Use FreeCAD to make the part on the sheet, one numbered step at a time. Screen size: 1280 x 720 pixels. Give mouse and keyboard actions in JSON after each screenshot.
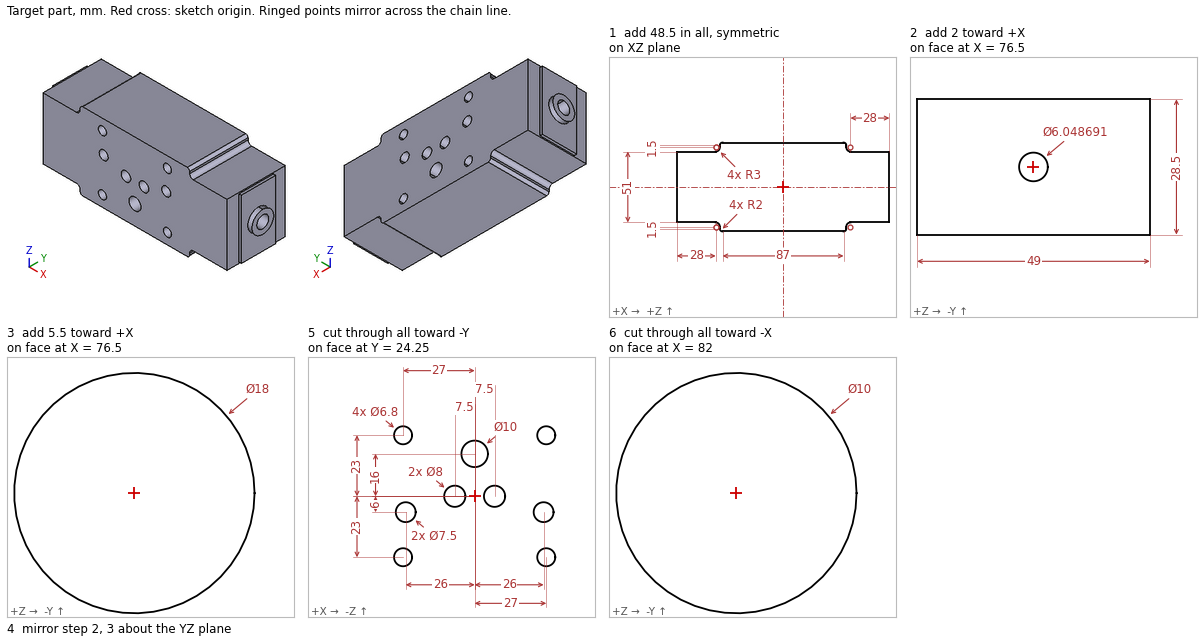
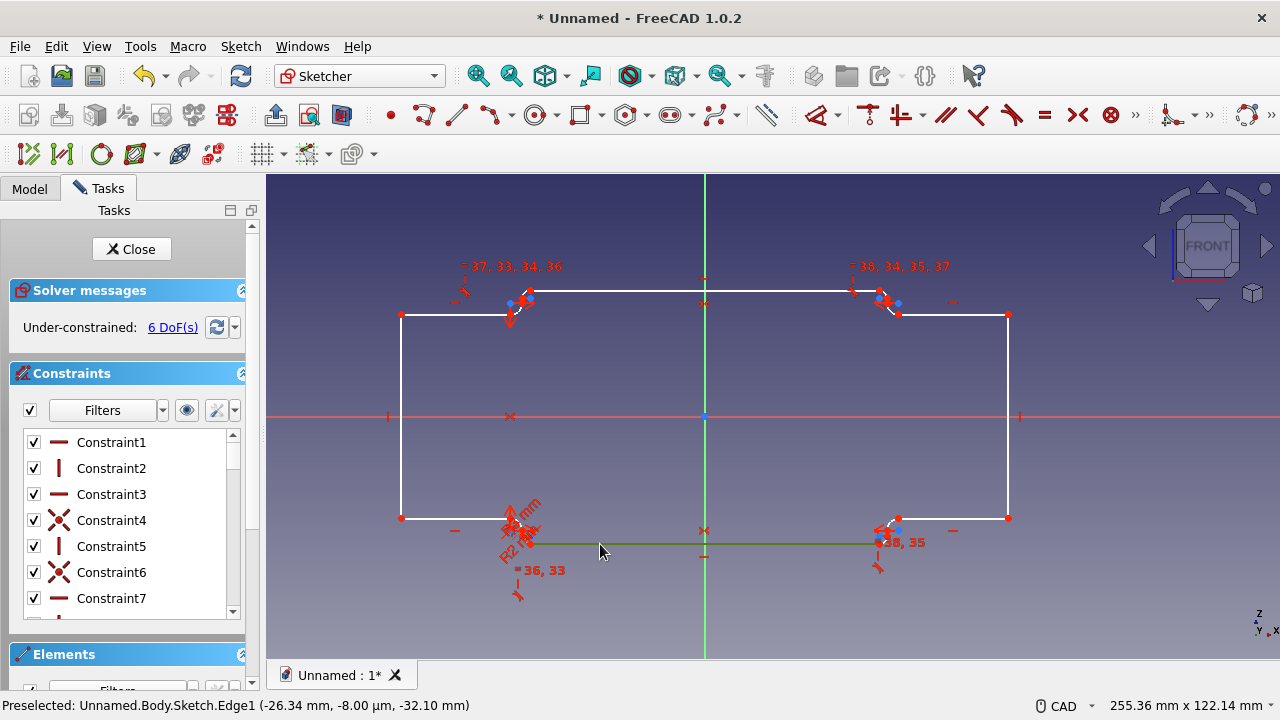
{"action": "key", "text": "l"}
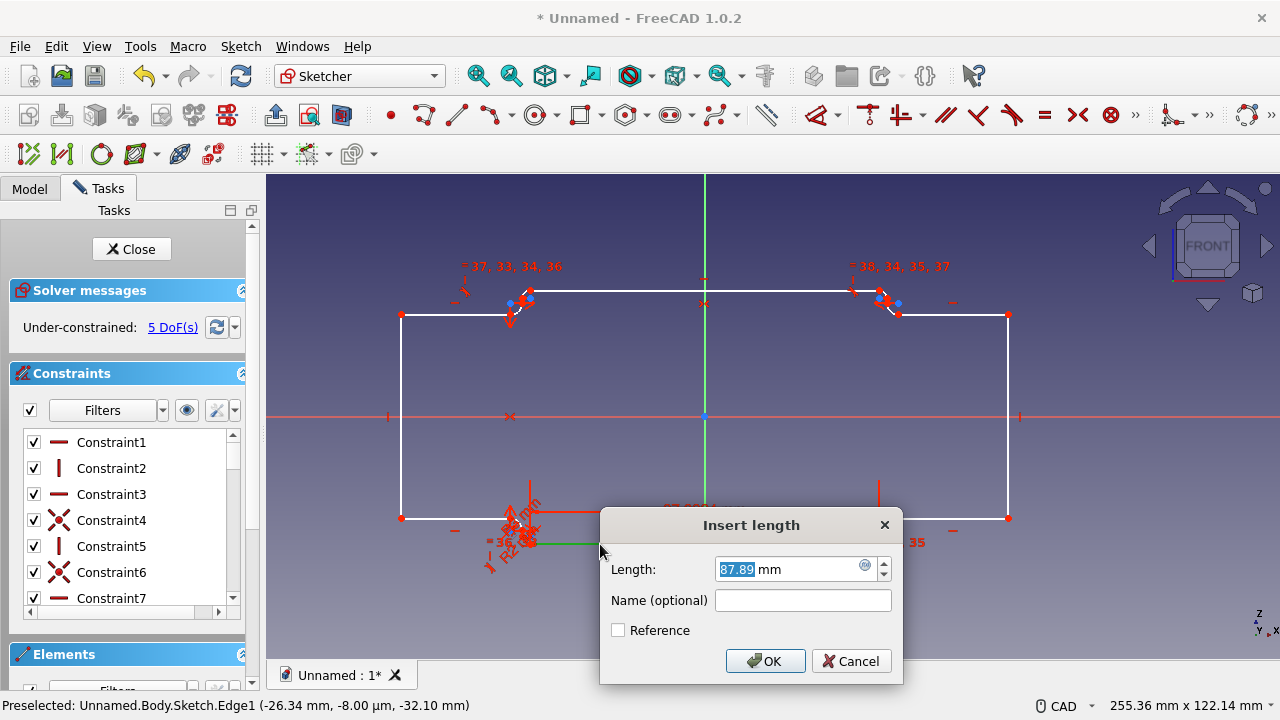
{"action": "type", "text": "87"}
{"action": "key", "text": "Return"}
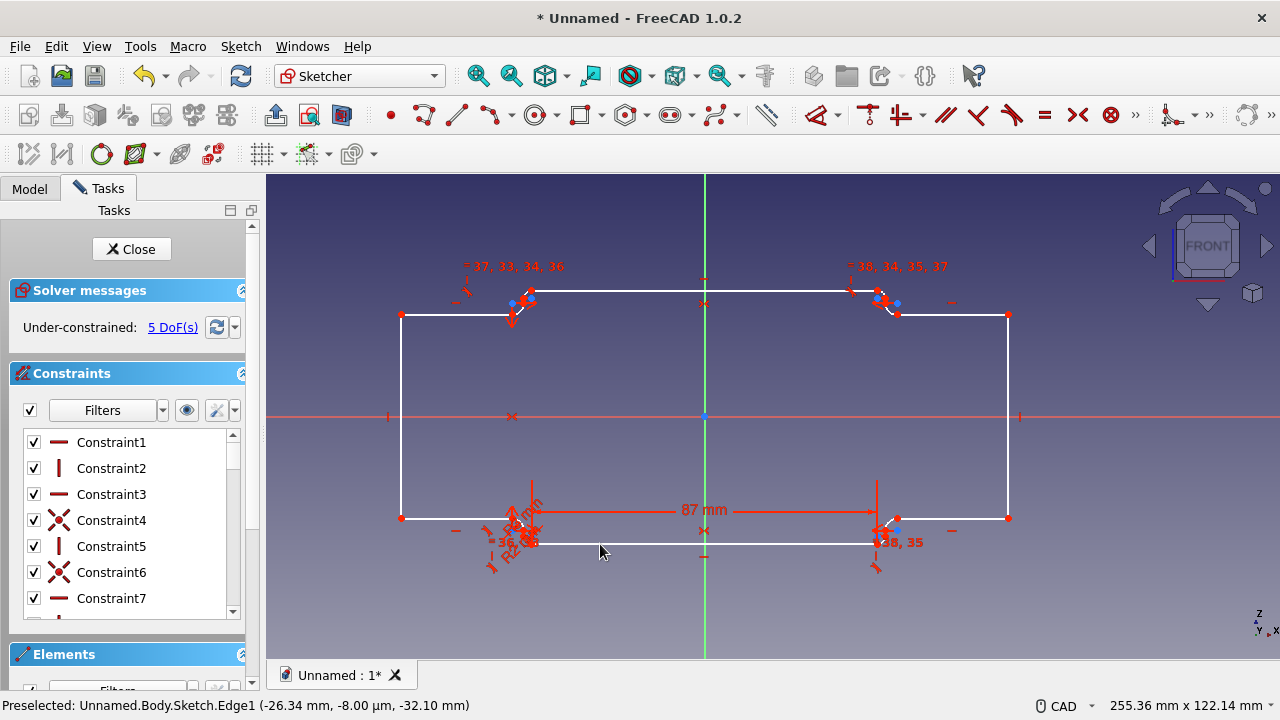
{"action": "left_click", "coordinate": [479, 519]}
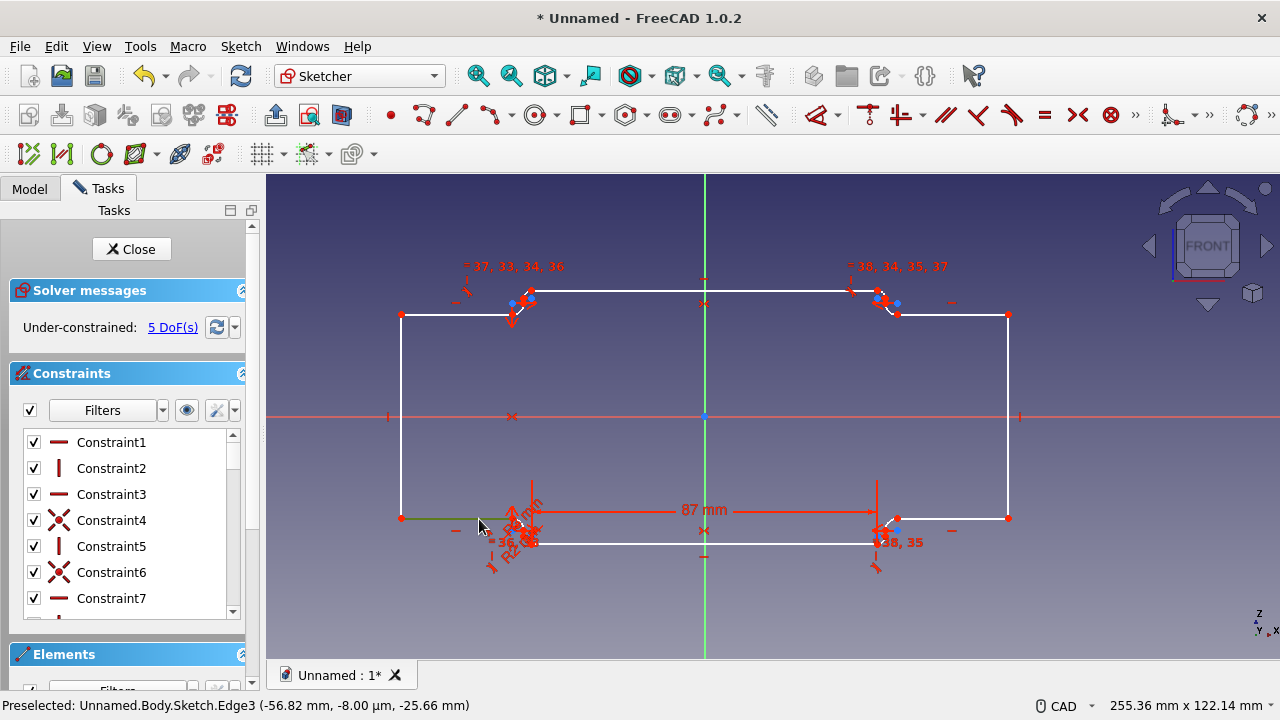
{"action": "key", "text": "l"}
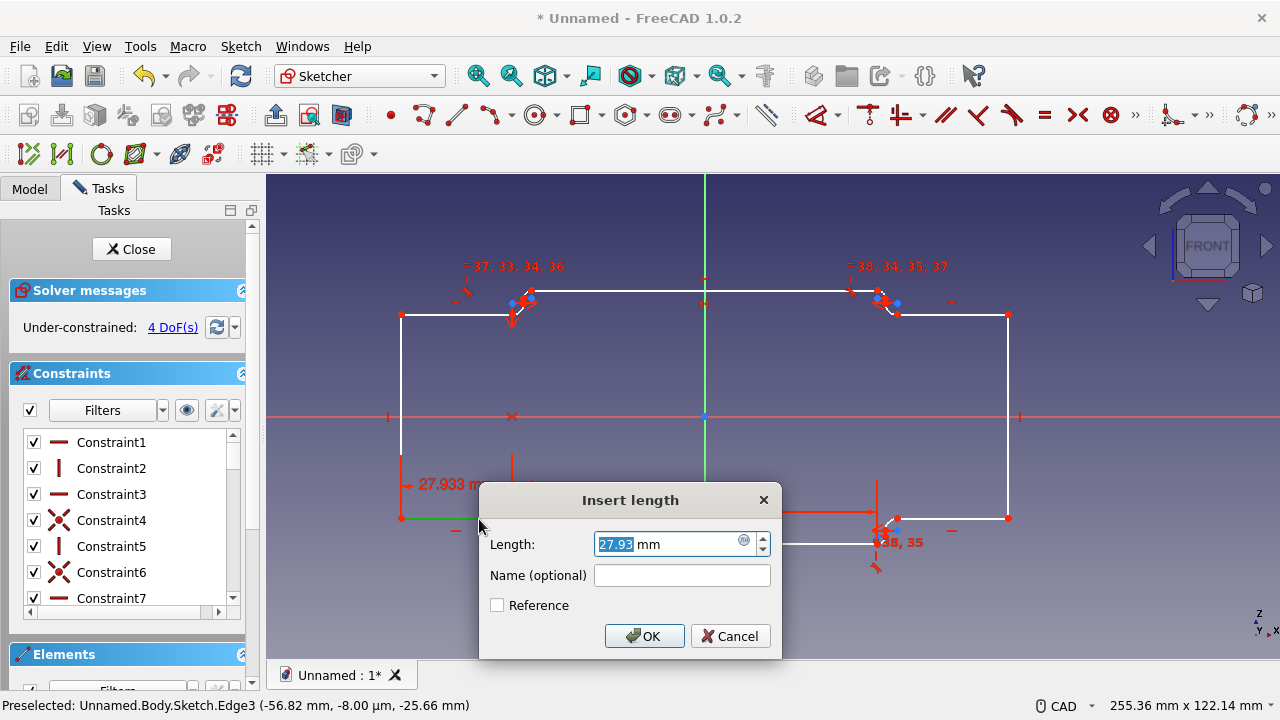
{"action": "type", "text": "28"}
{"action": "key", "text": "Return"}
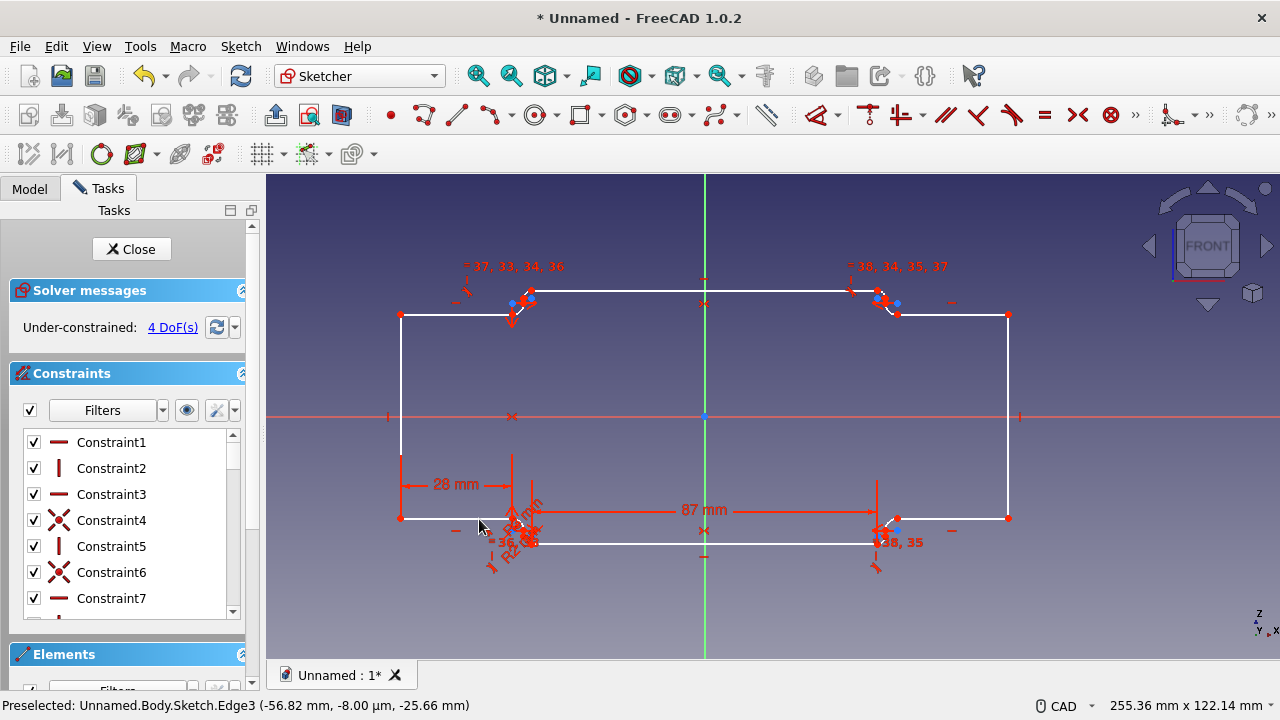
{"action": "left_click", "coordinate": [401, 458]}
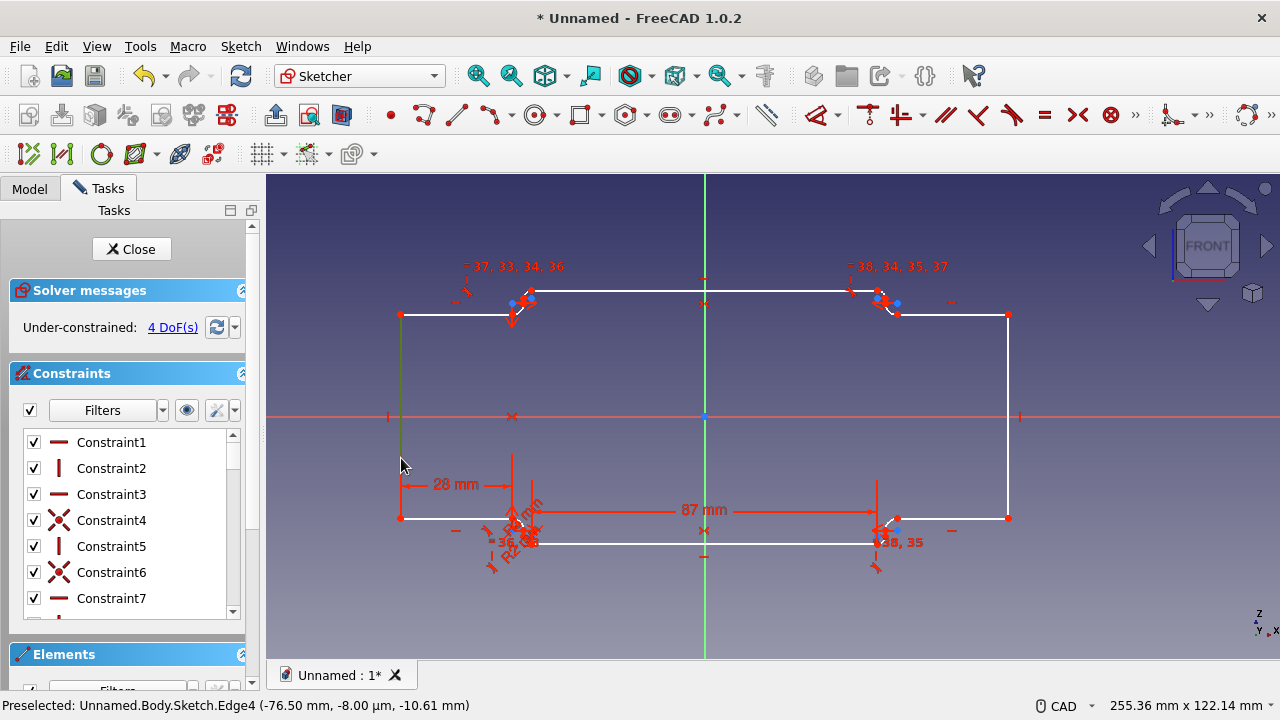
{"action": "left_click", "coordinate": [838, 116]}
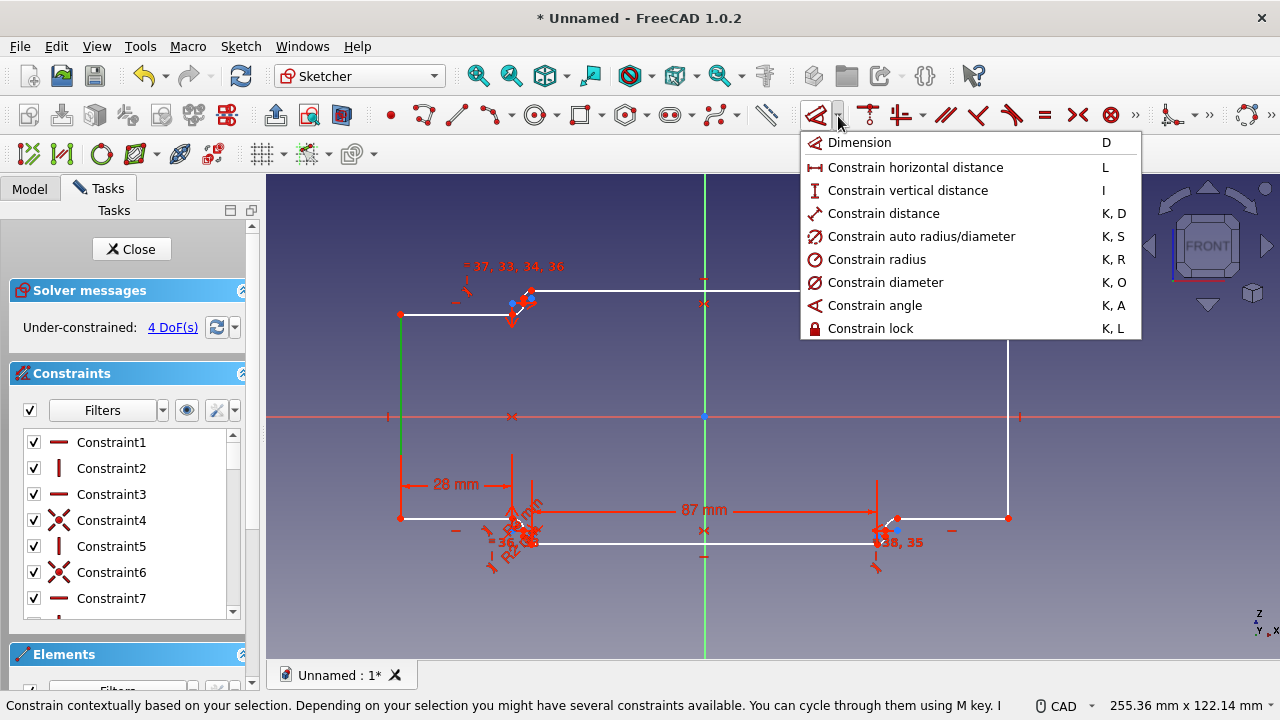
{"action": "left_click", "coordinate": [971, 190]}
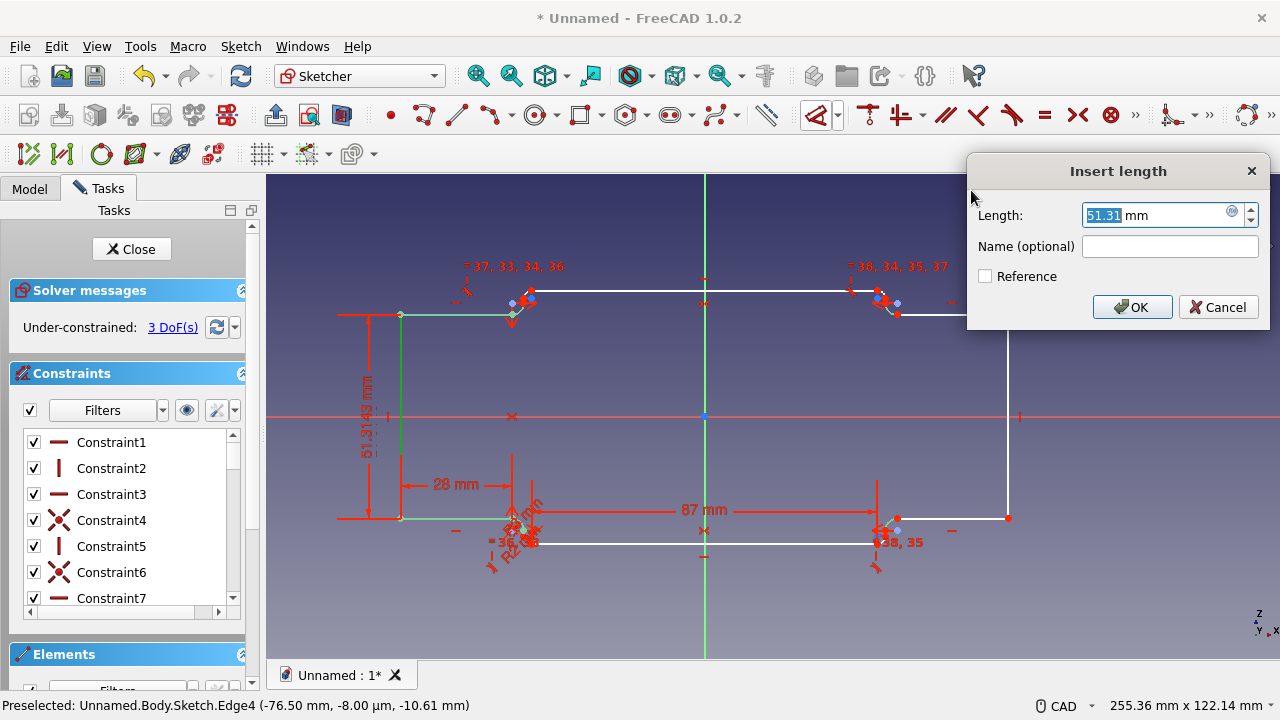
{"action": "type", "text": "51"}
{"action": "key", "text": "Return"}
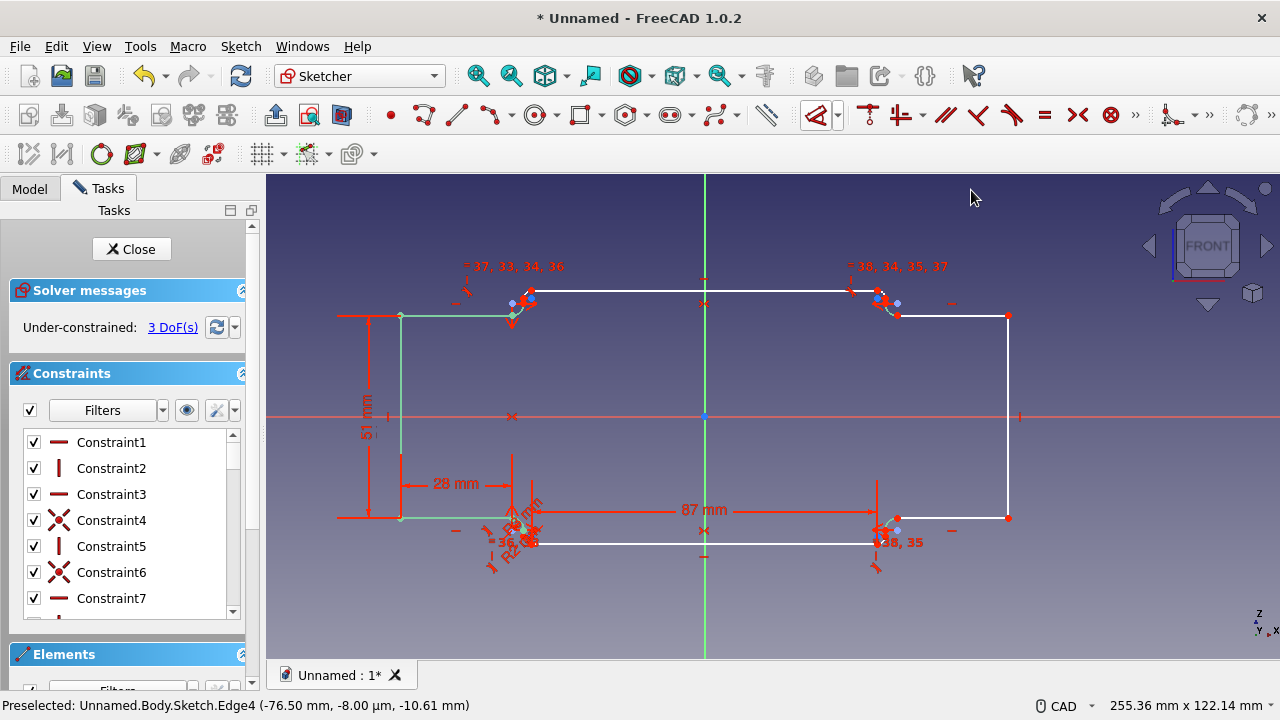
{"action": "left_click", "coordinate": [931, 316]}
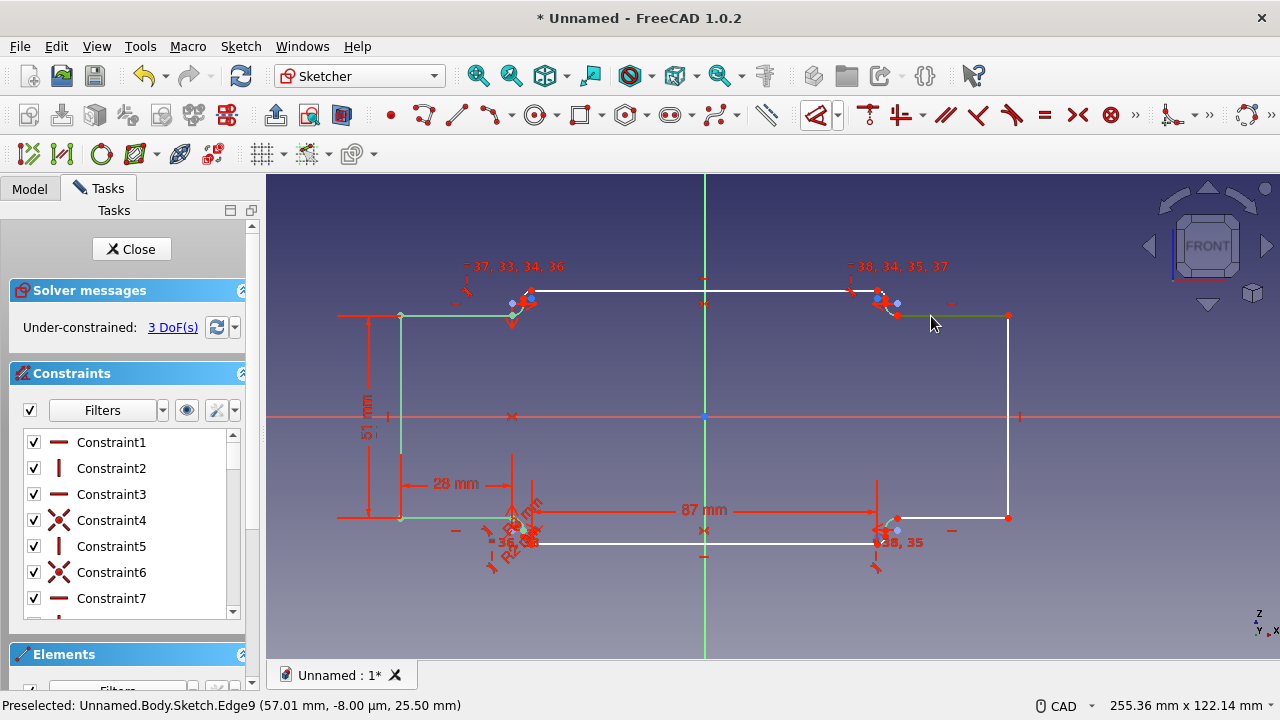
{"action": "left_click", "coordinate": [838, 116]}